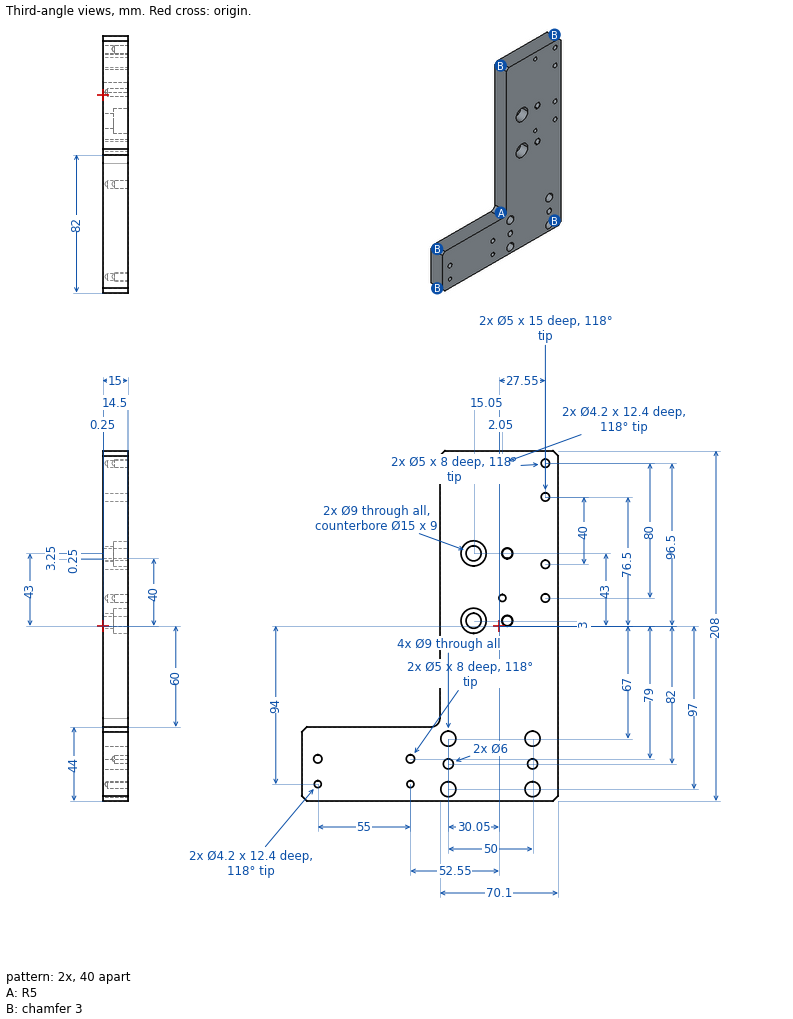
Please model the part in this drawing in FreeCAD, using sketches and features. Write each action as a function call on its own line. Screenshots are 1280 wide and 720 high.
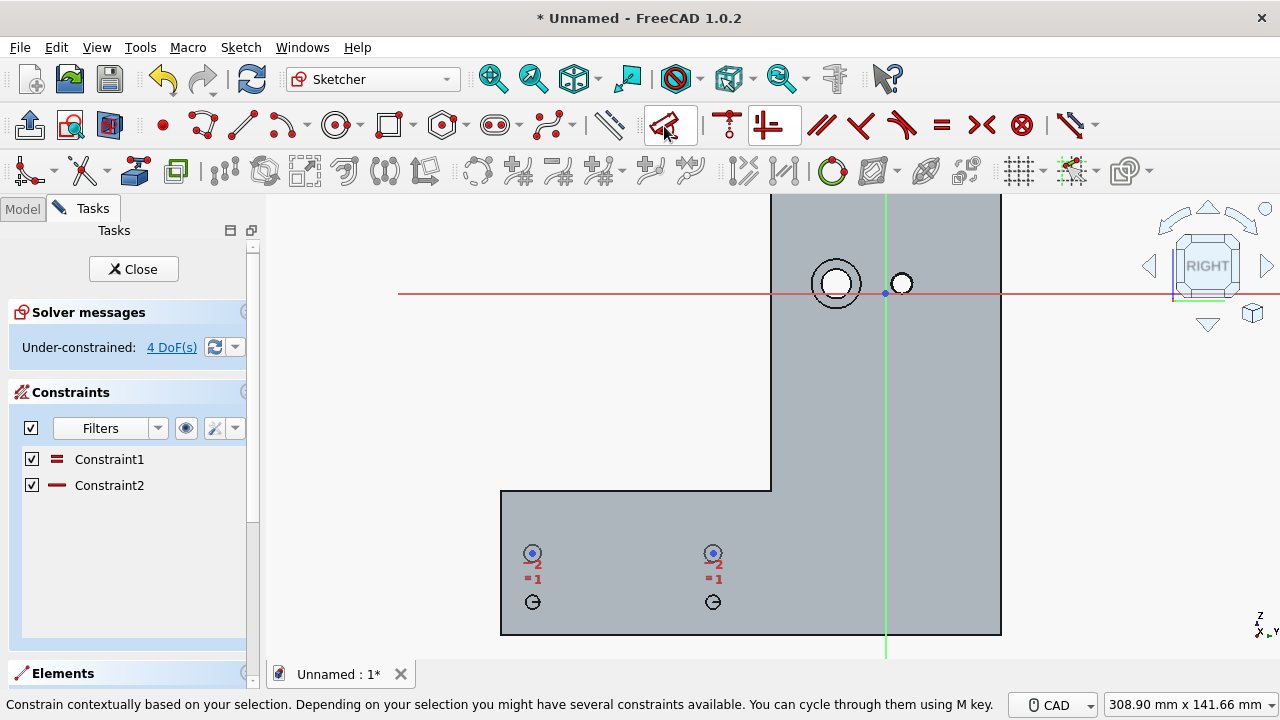
scroll(719, 547, up, 5)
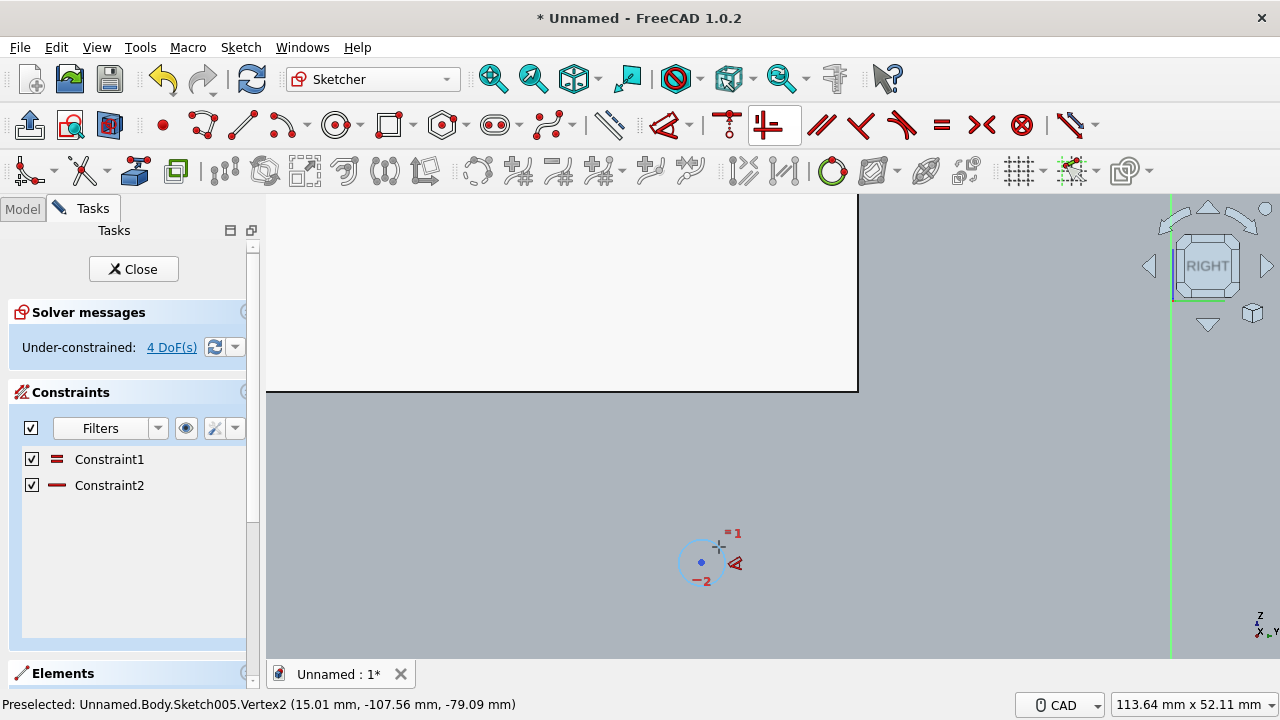
click(718, 546)
click(740, 523)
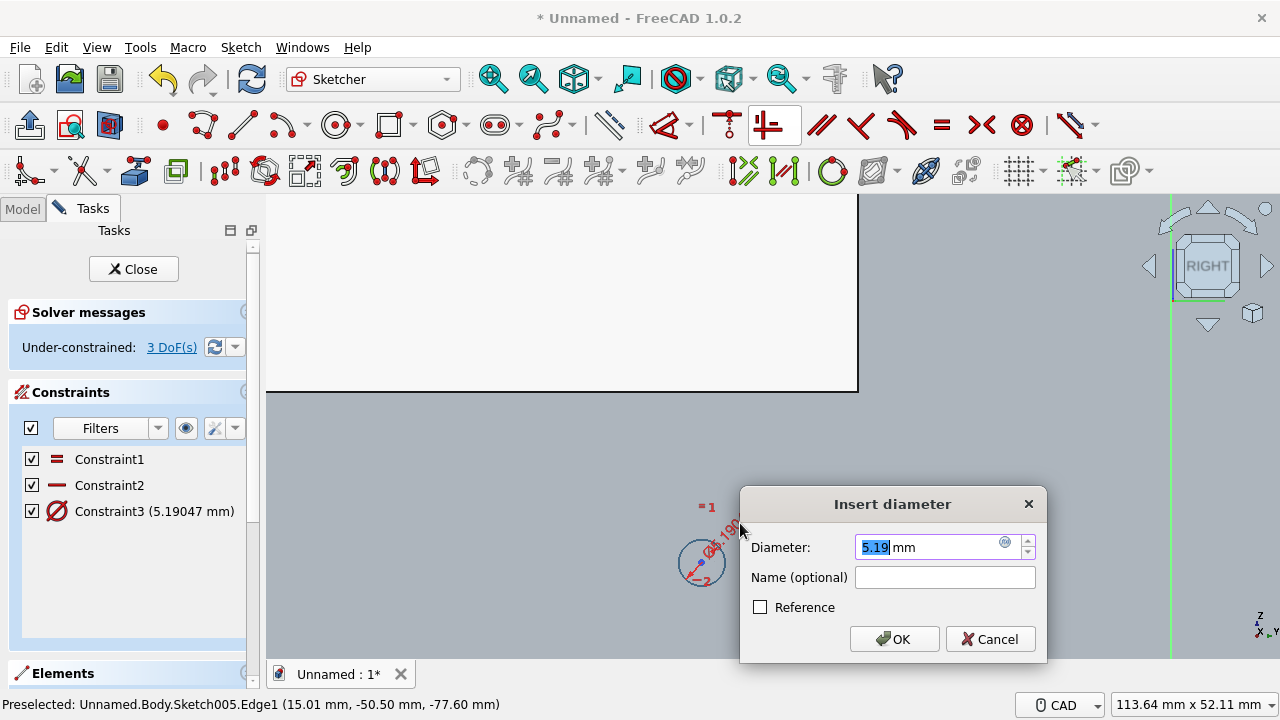
text(5)
key(Return)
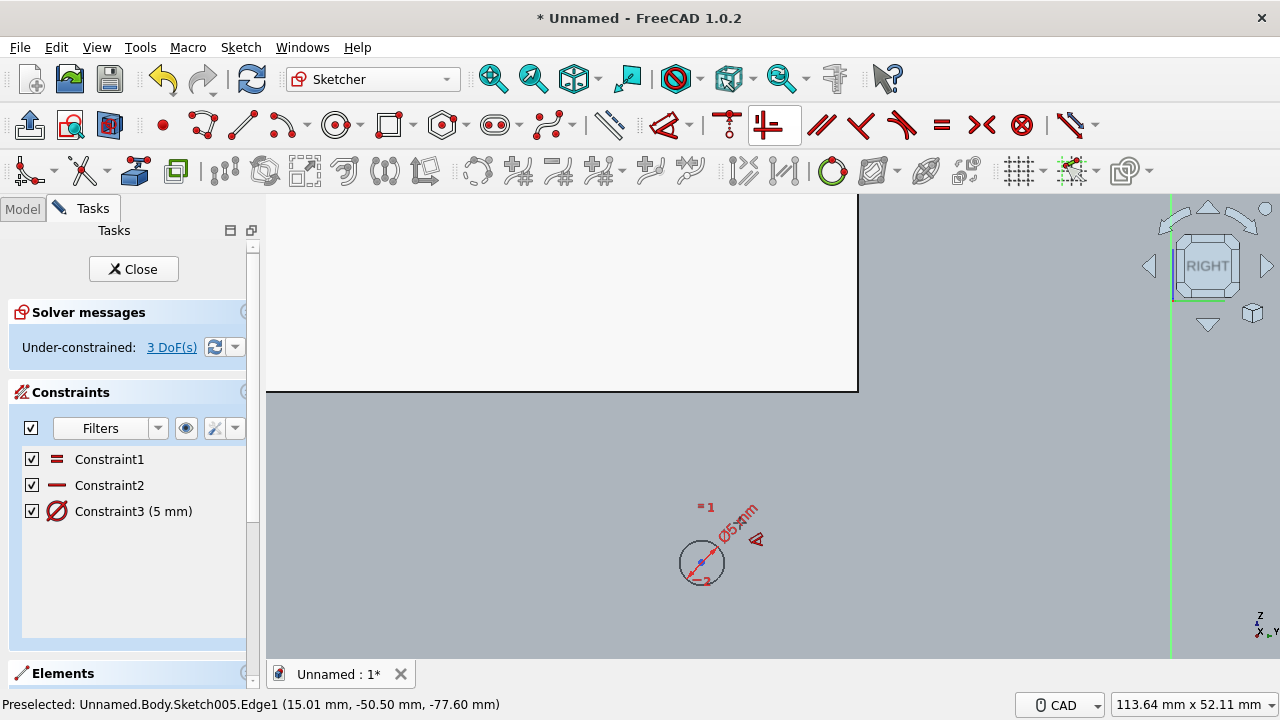
click(702, 563)
click(668, 392)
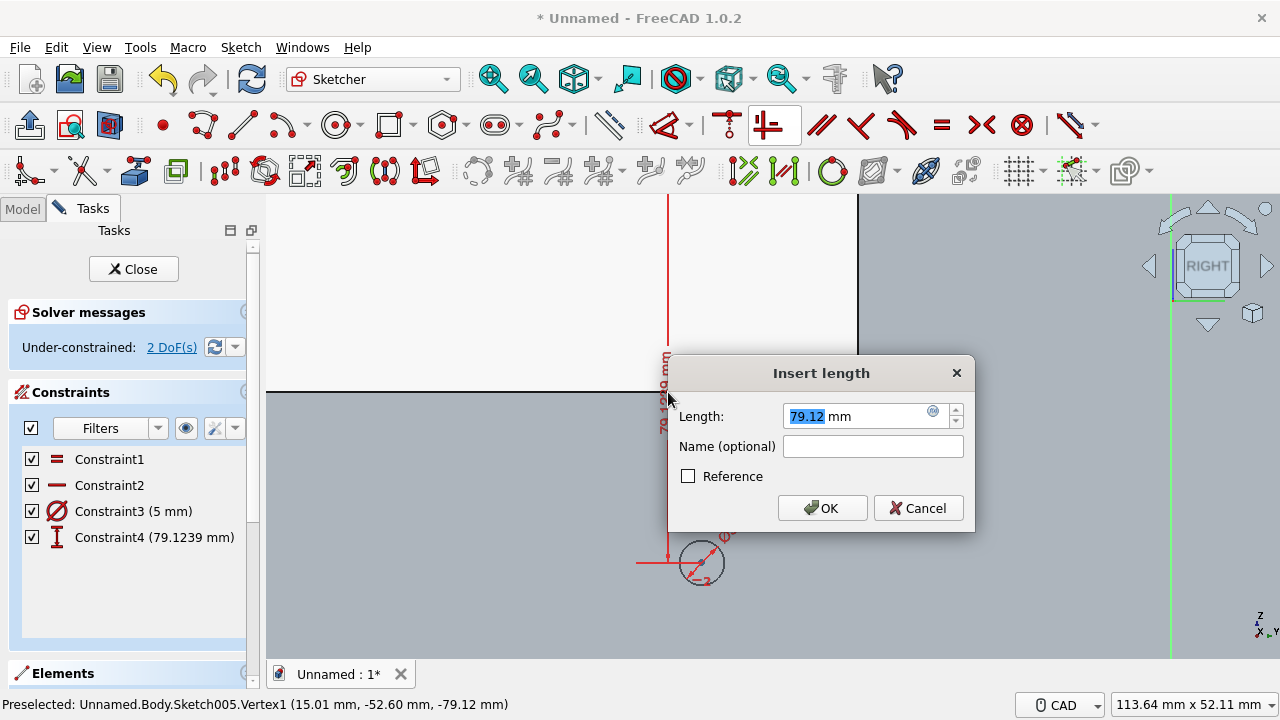
text(79)
key(Return)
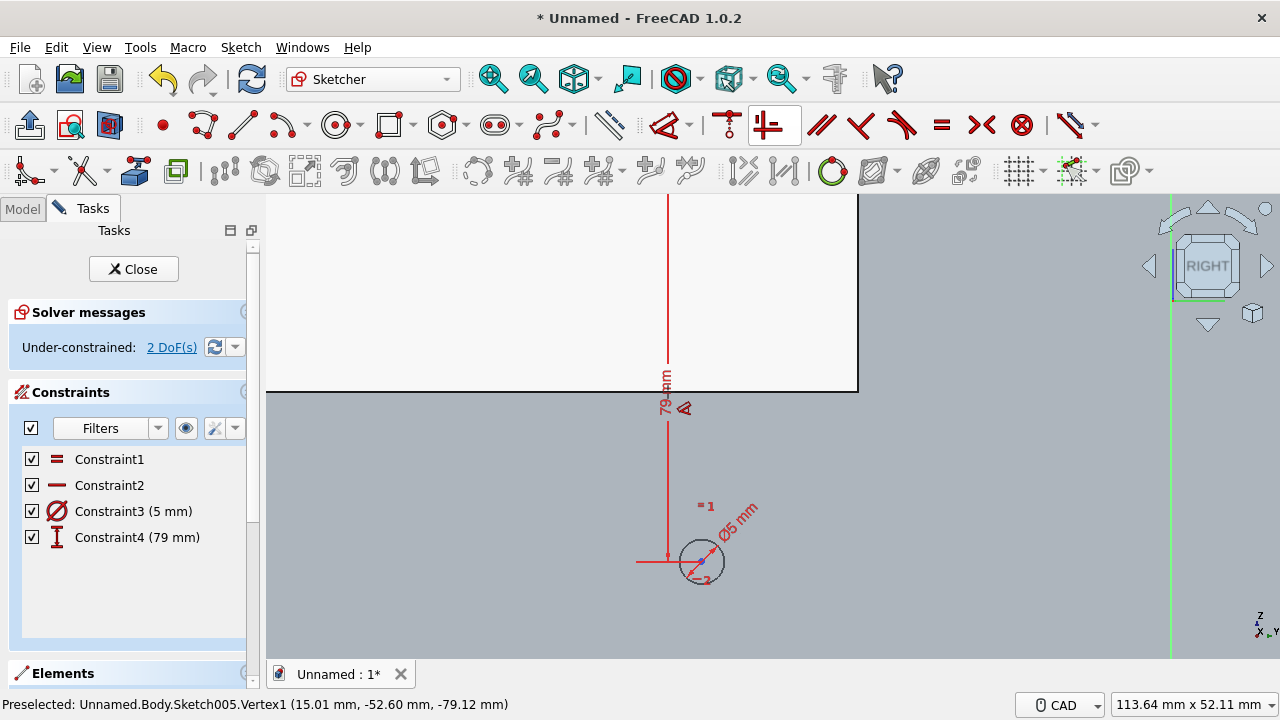
click(702, 562)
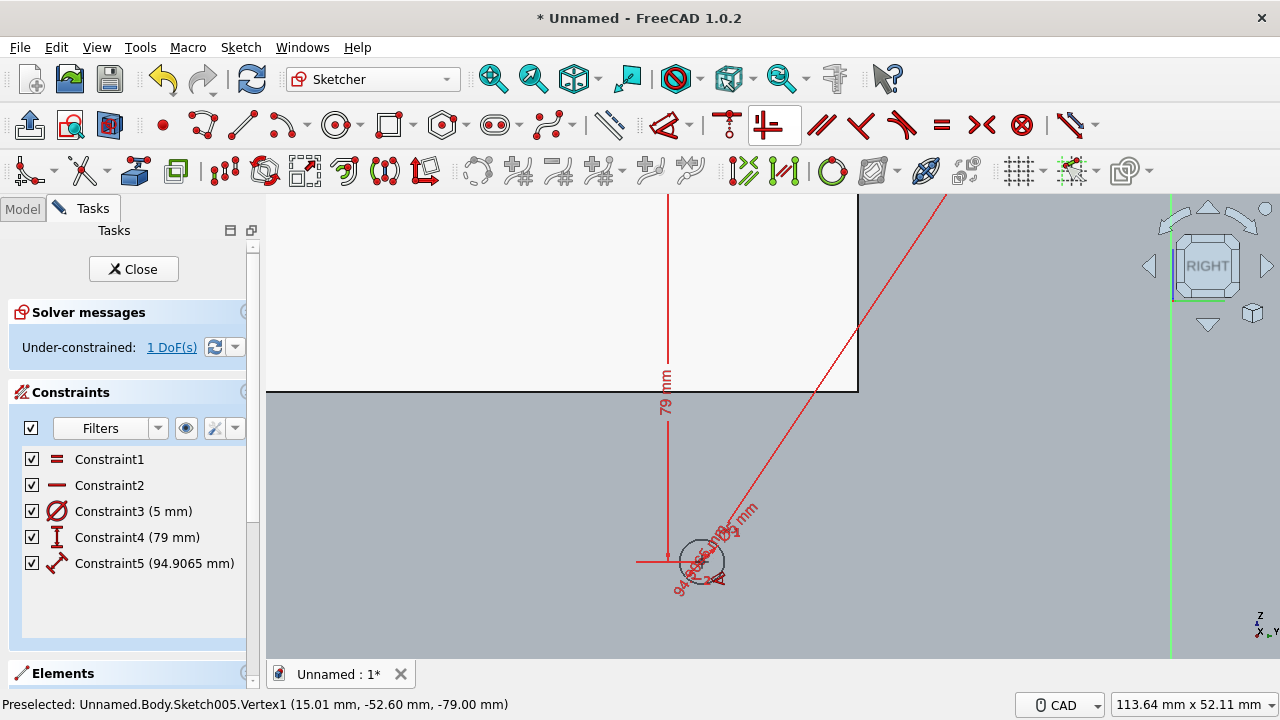
scroll(719, 546, down, 5)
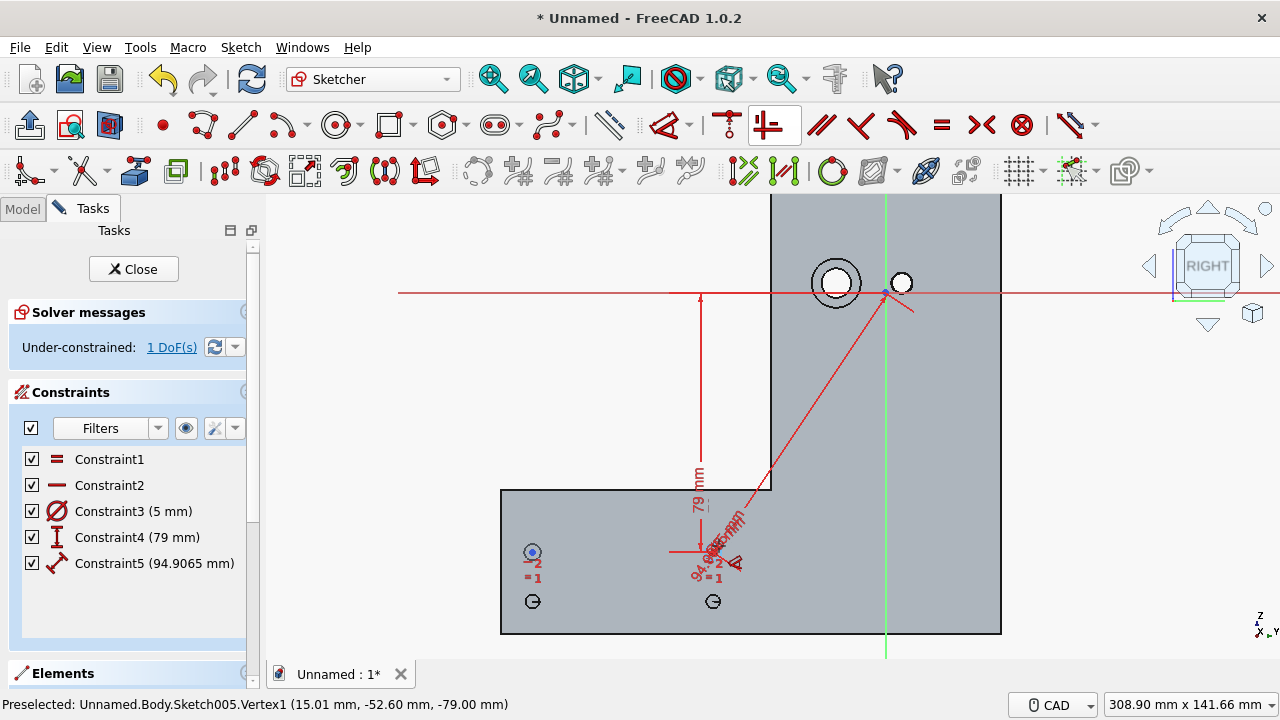
click(533, 552)
click(623, 586)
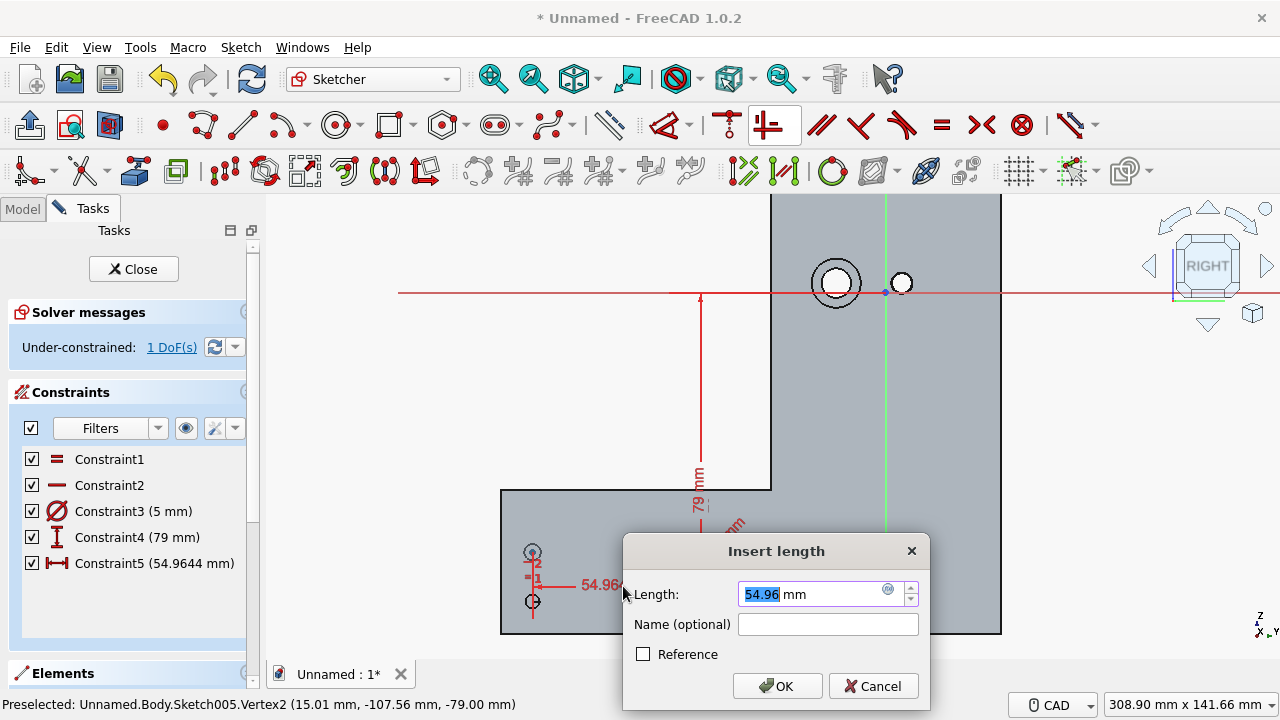
text(55)
key(Return)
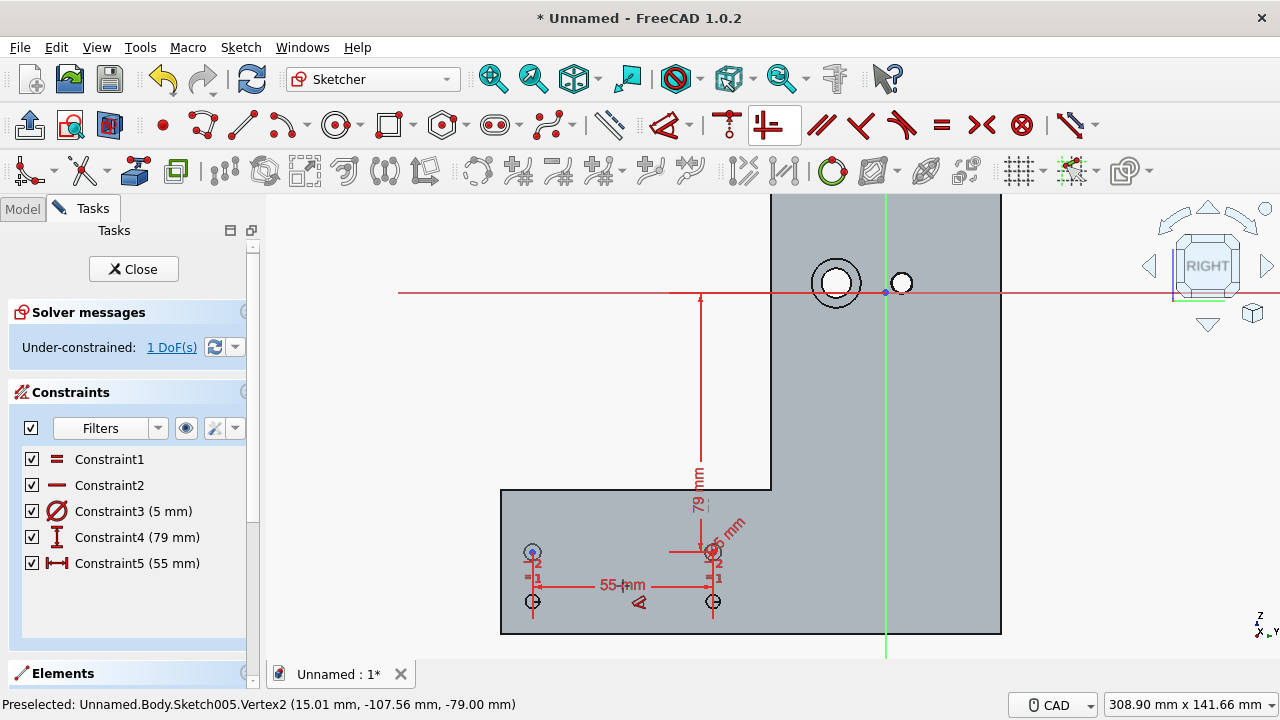
click(713, 552)
click(799, 259)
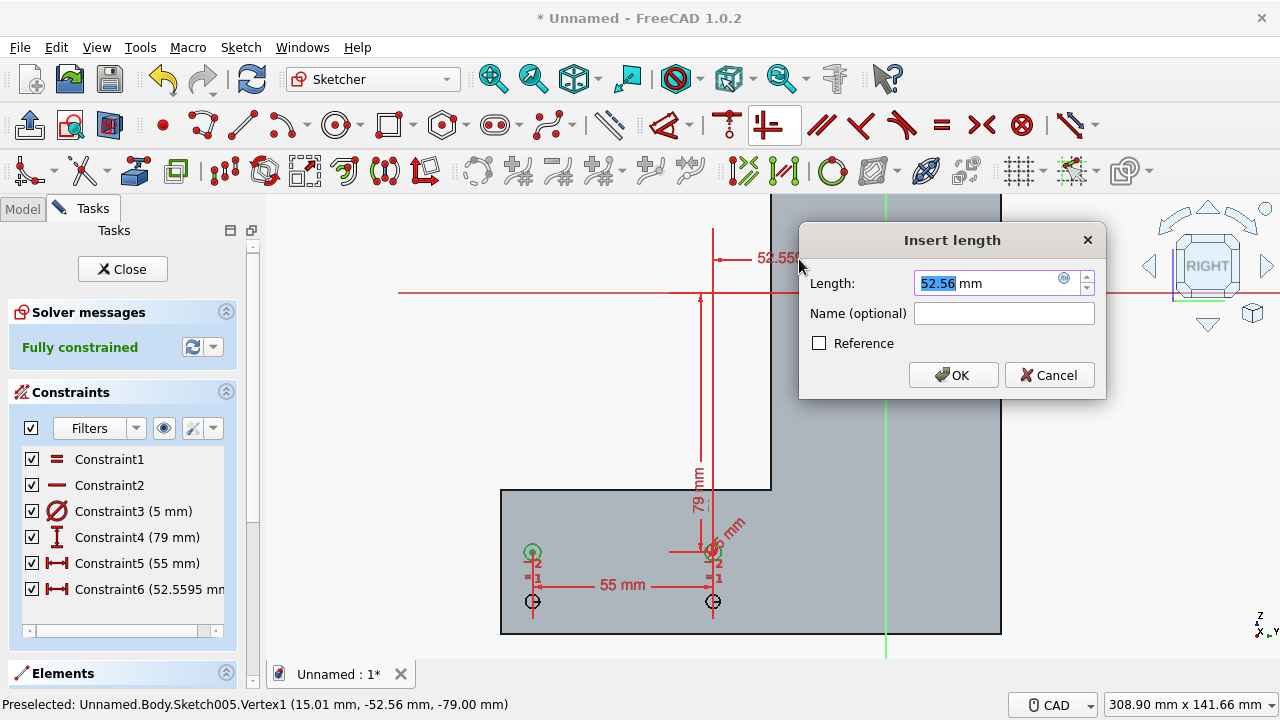
text(52.55)
key(Return)
key(Escape)